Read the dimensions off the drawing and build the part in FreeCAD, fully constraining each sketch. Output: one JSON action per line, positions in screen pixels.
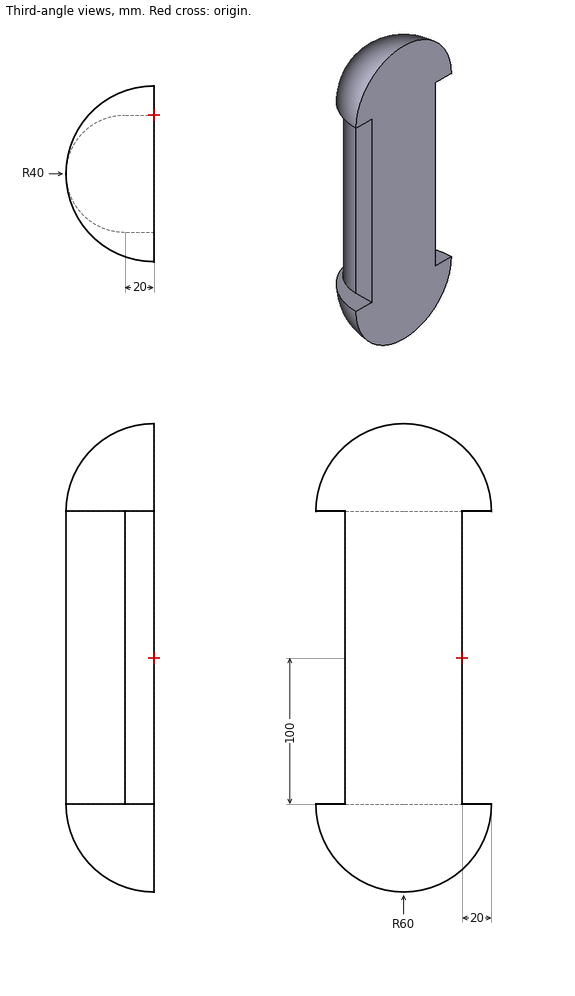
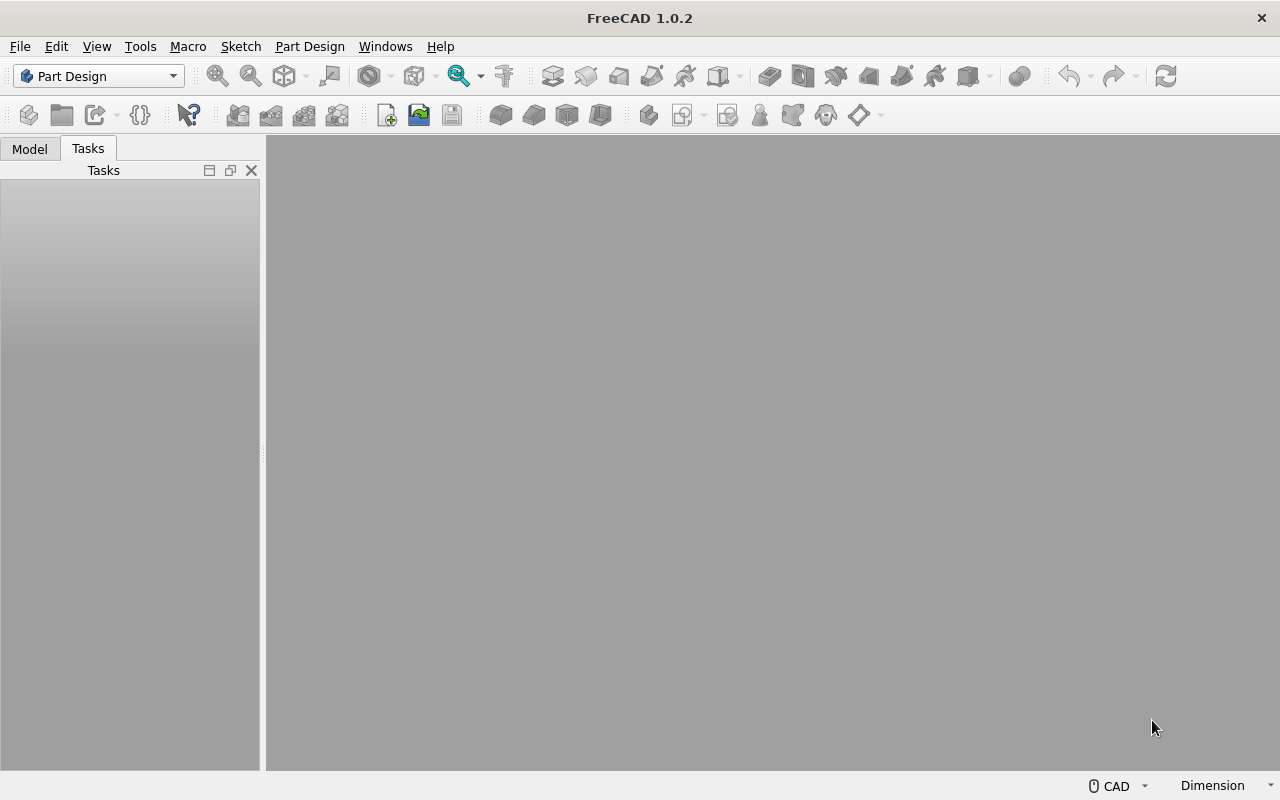
{"action": "key", "text": "ctrl+n"}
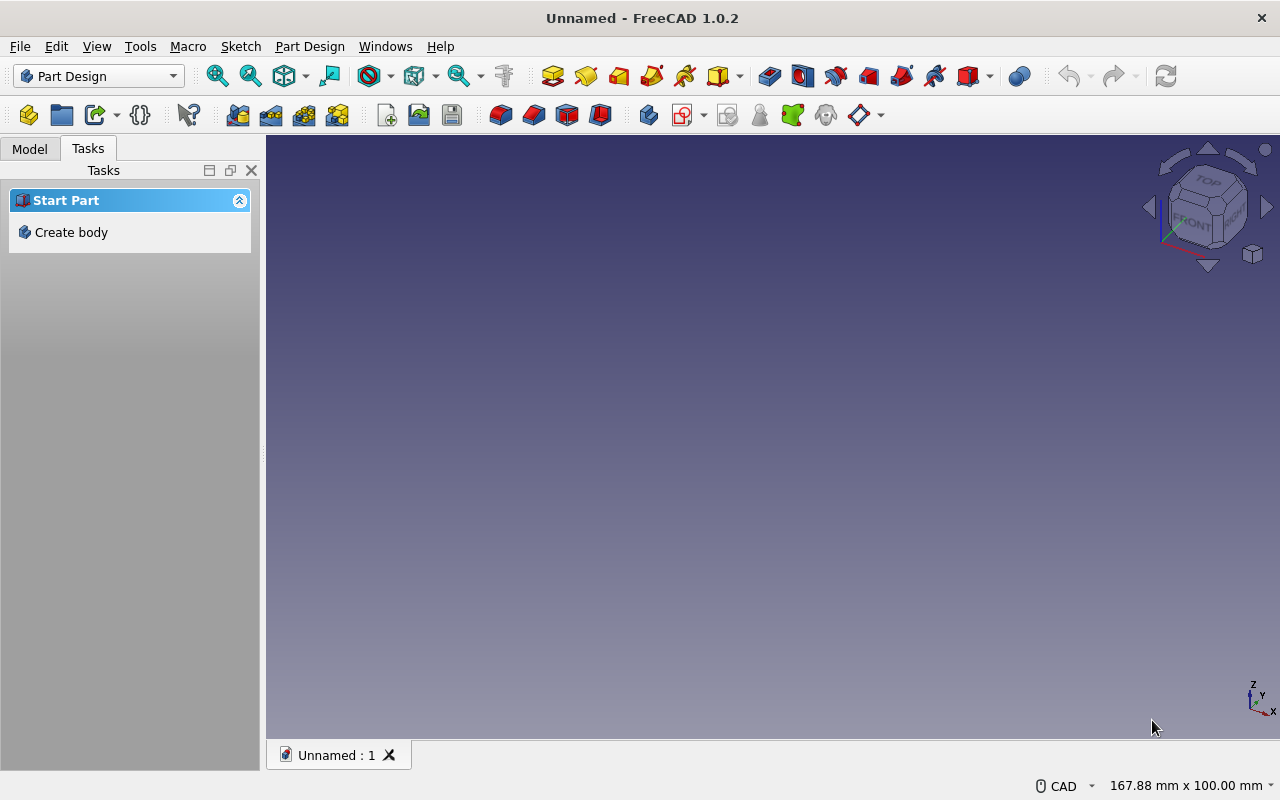
{"action": "left_click", "coordinate": [682, 116]}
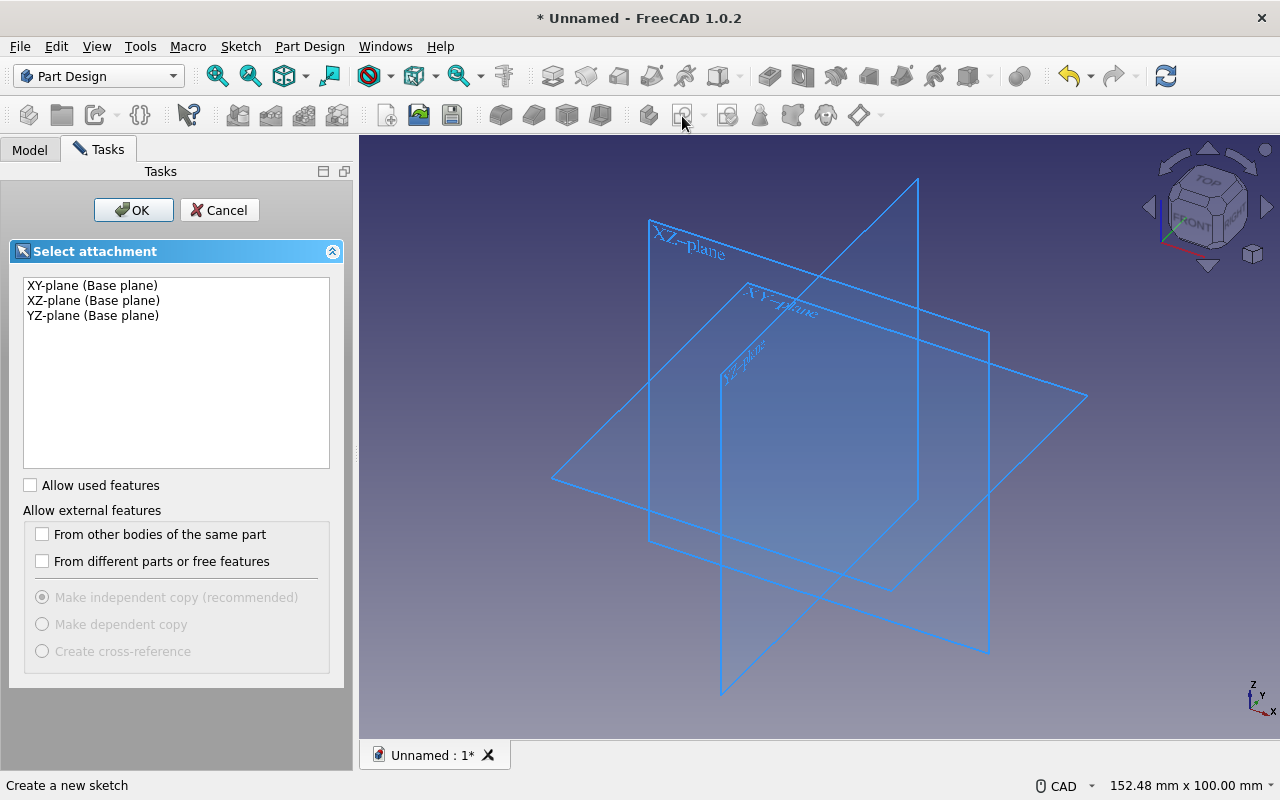
{"action": "left_click", "coordinate": [84, 286]}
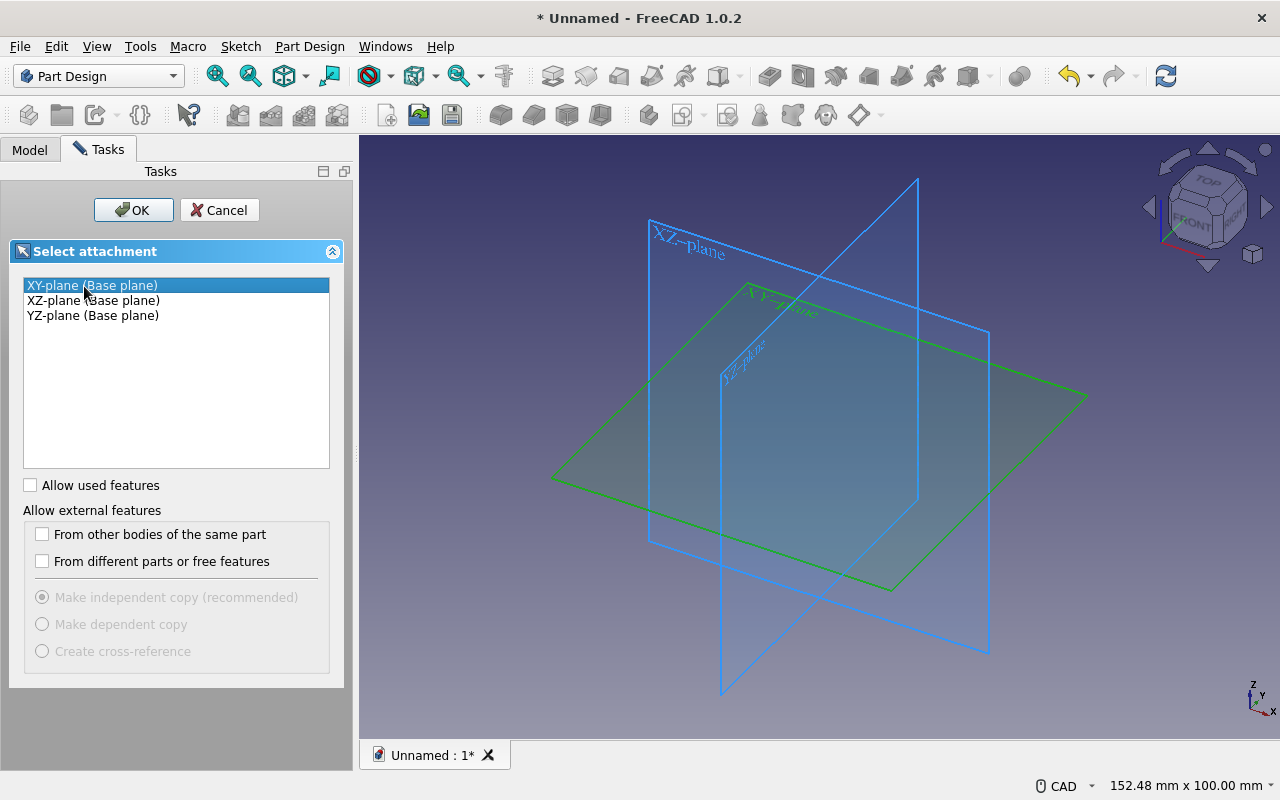
{"action": "left_click", "coordinate": [134, 210]}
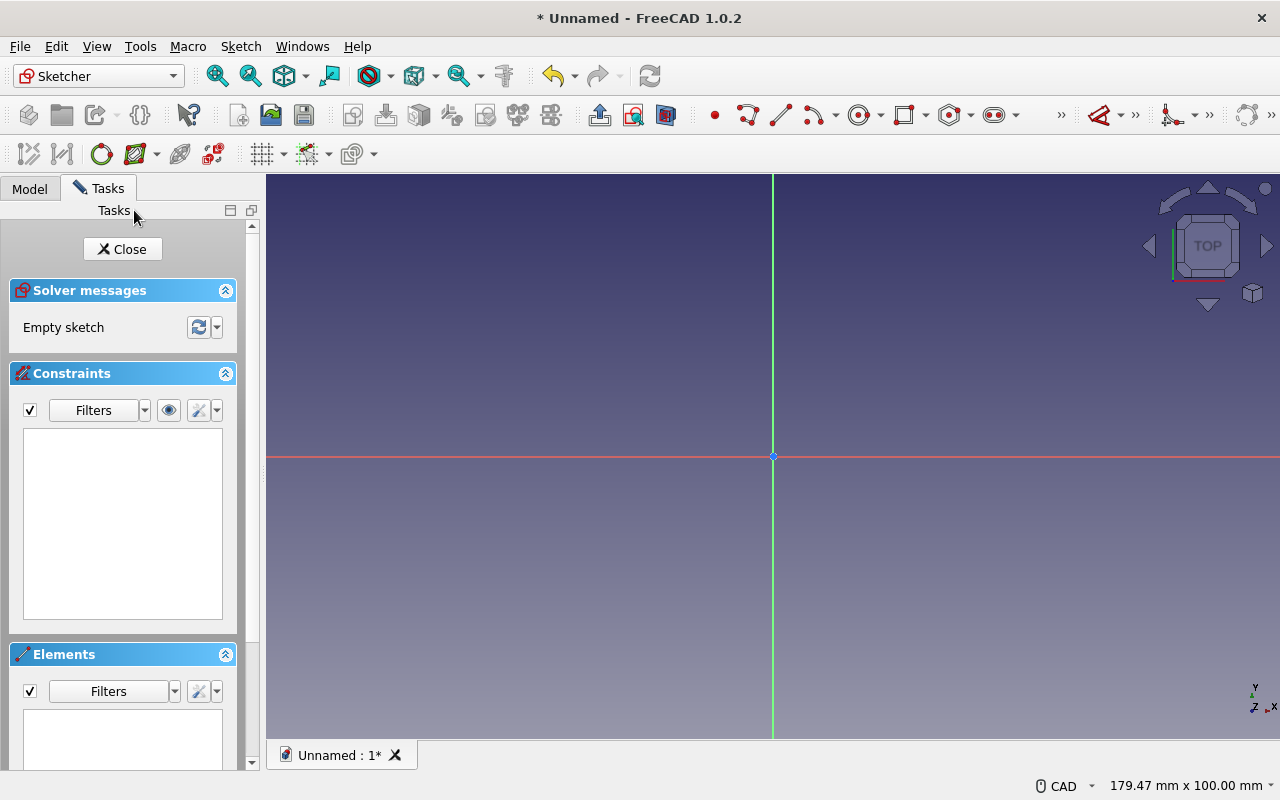
{"action": "scroll", "coordinate": [910, 202], "scroll_direction": "down", "scroll_amount": 2}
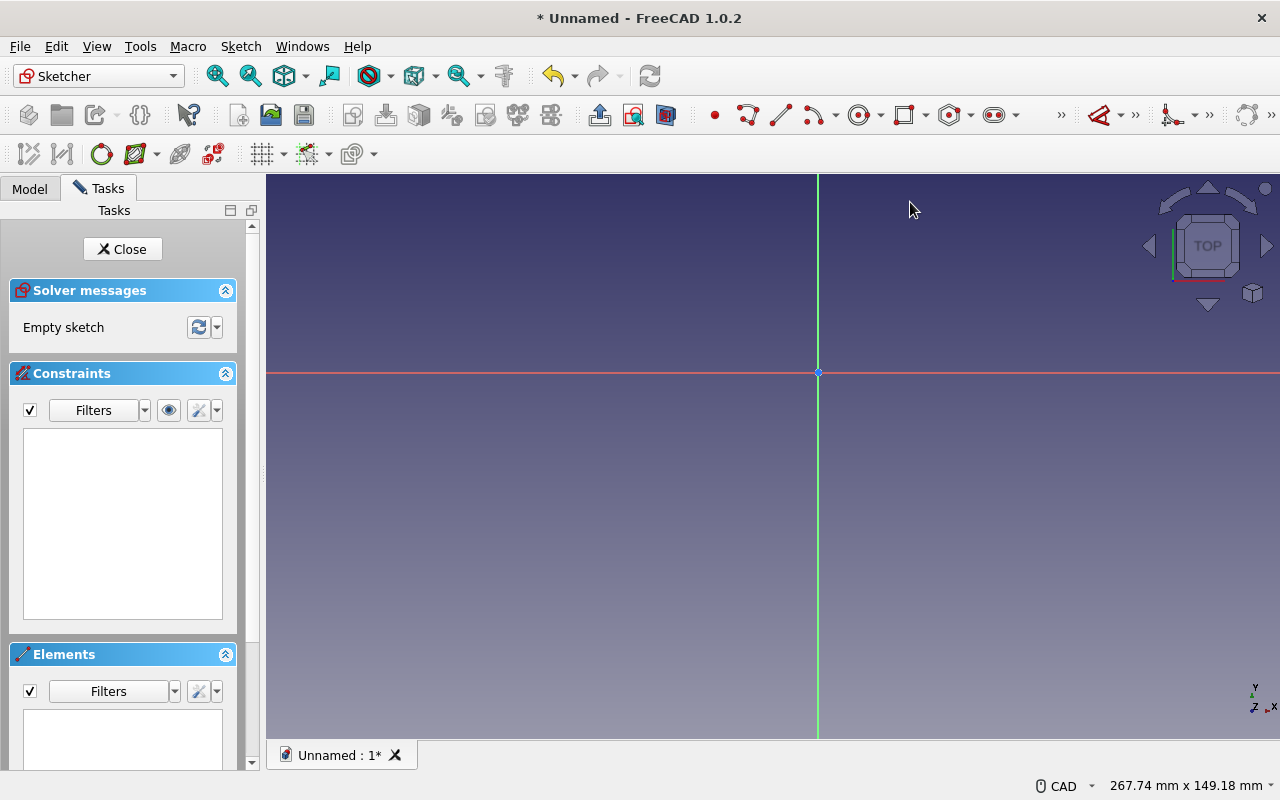
{"action": "left_click", "coordinate": [748, 116]}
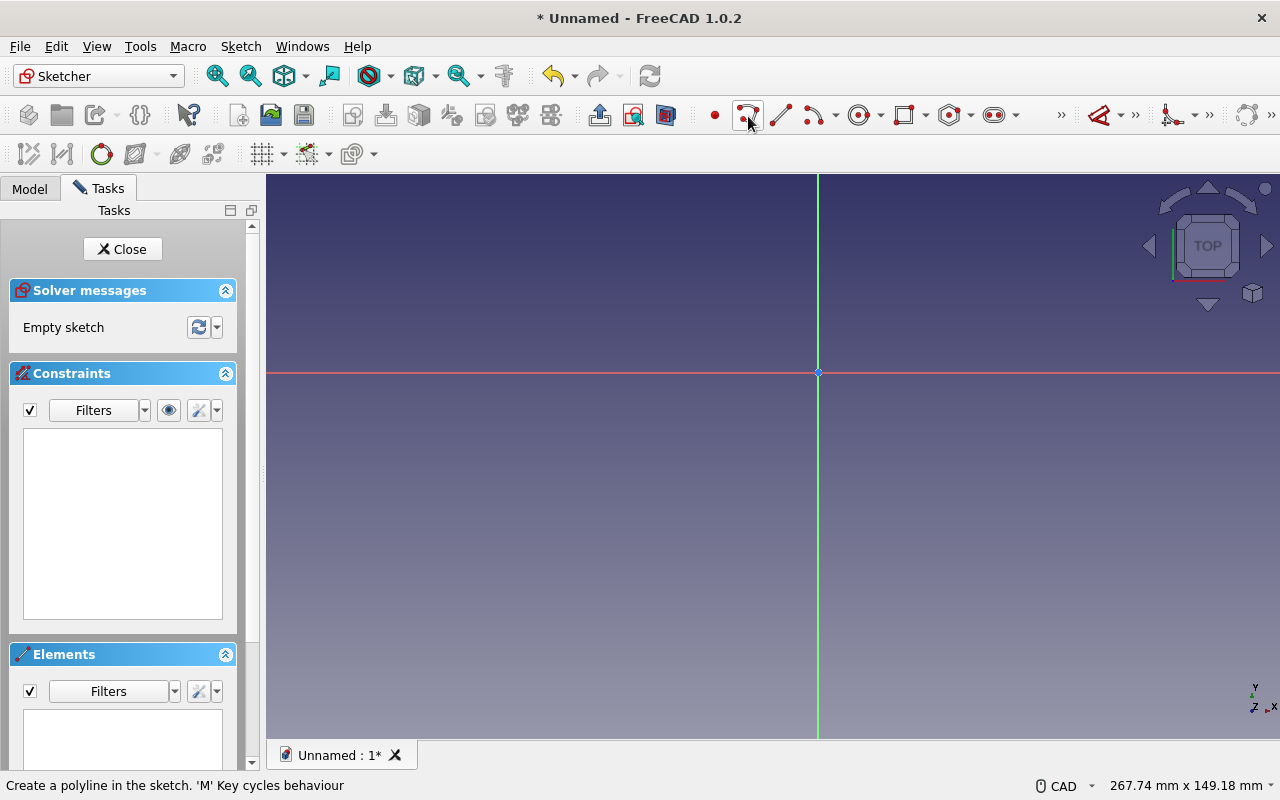
{"action": "left_click", "coordinate": [743, 676]}
{"action": "left_click", "coordinate": [818, 676]}
{"action": "left_click", "coordinate": [818, 373]}
{"action": "left_click", "coordinate": [743, 382]}
{"action": "right_click", "coordinate": [743, 382]}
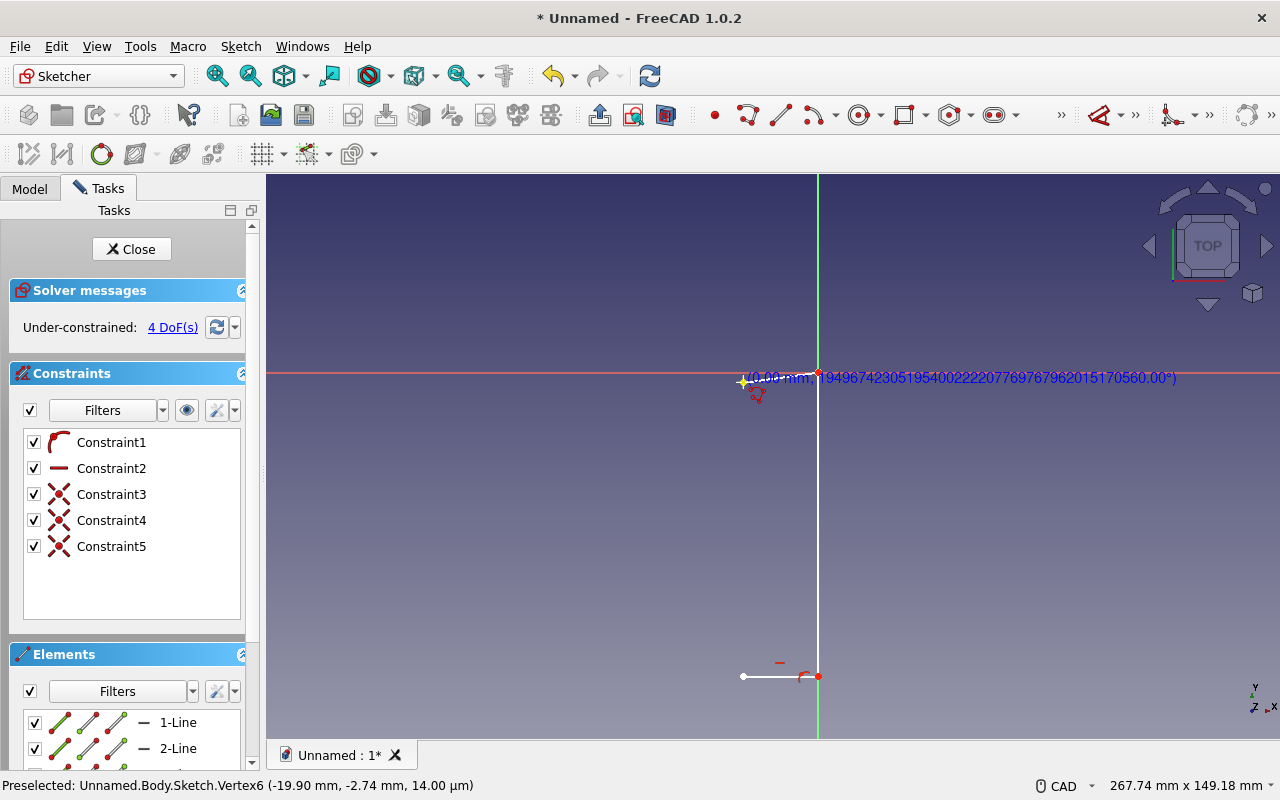
{"action": "key", "text": "g 3 a"}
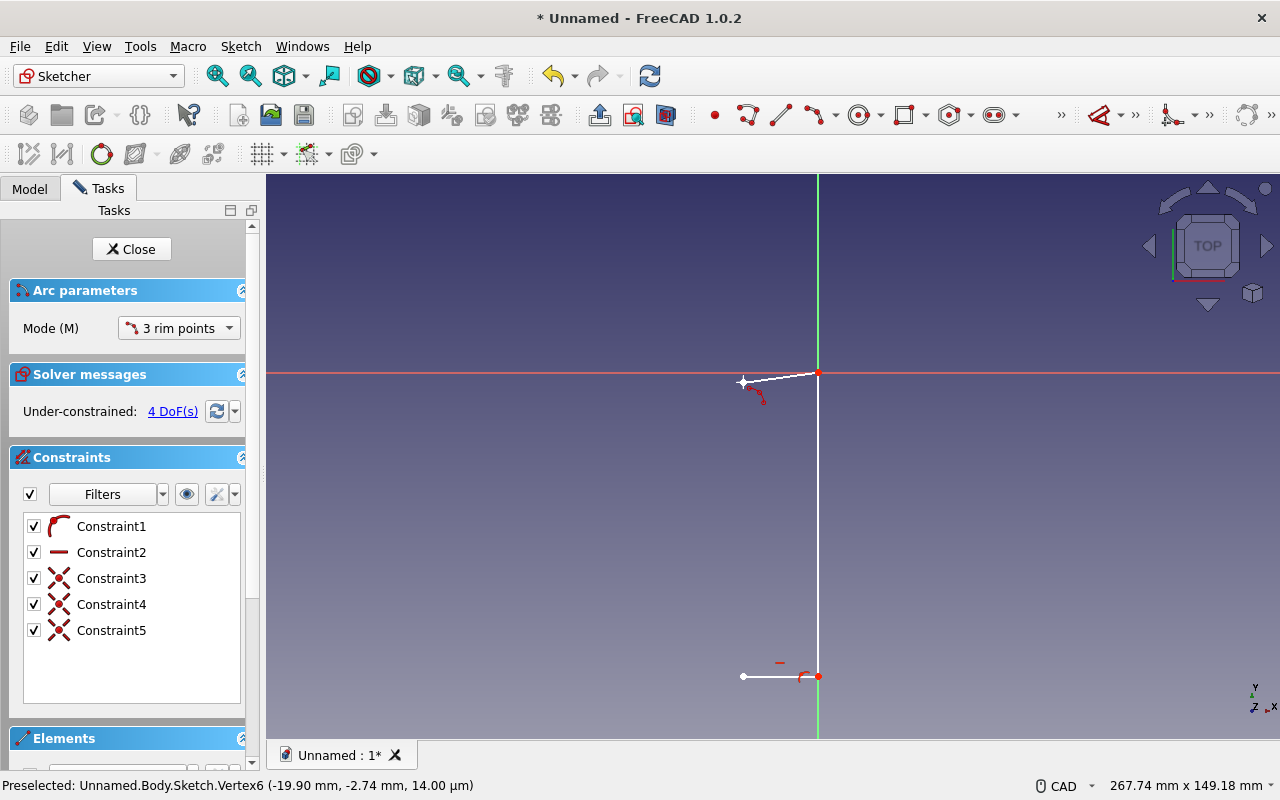
{"action": "left_click", "coordinate": [743, 383]}
{"action": "left_click", "coordinate": [743, 677]}
{"action": "left_click", "coordinate": [591, 524]}
{"action": "key", "text": "Escape"}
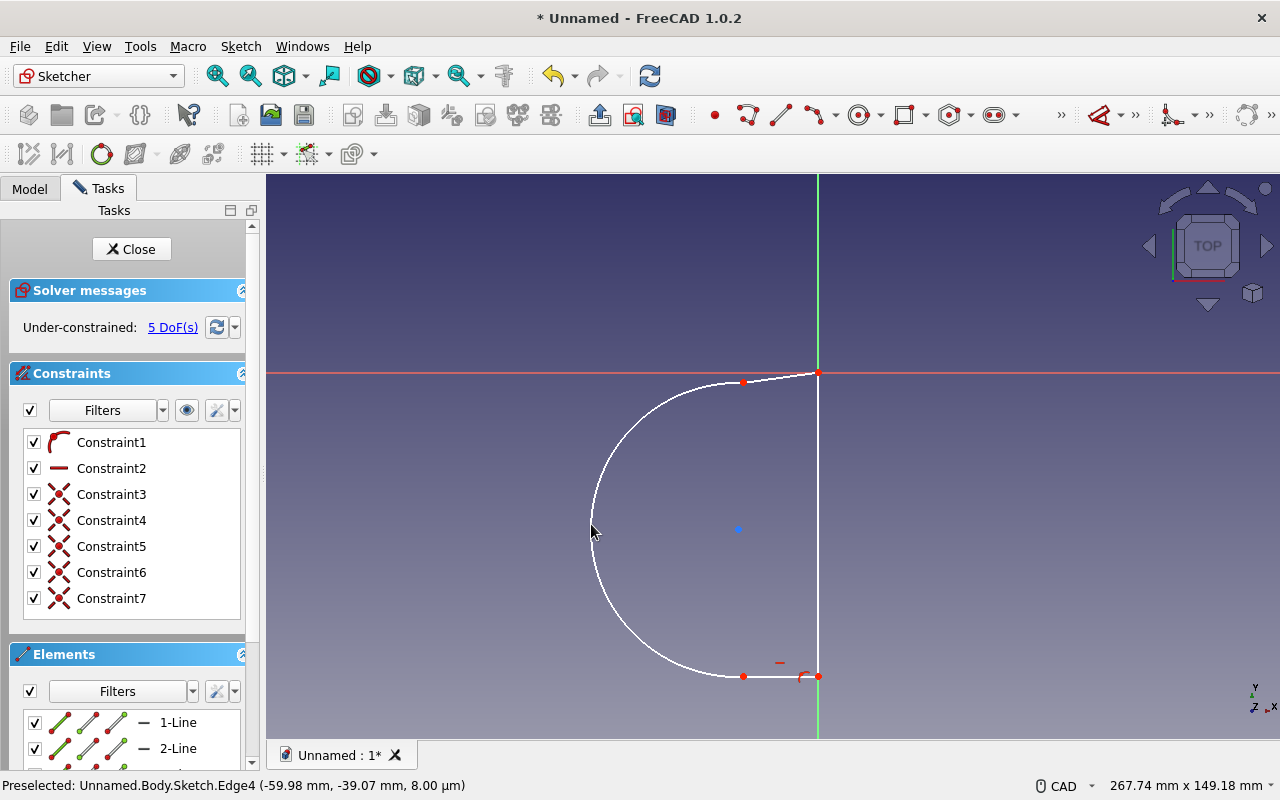
{"action": "left_click", "coordinate": [796, 376]}